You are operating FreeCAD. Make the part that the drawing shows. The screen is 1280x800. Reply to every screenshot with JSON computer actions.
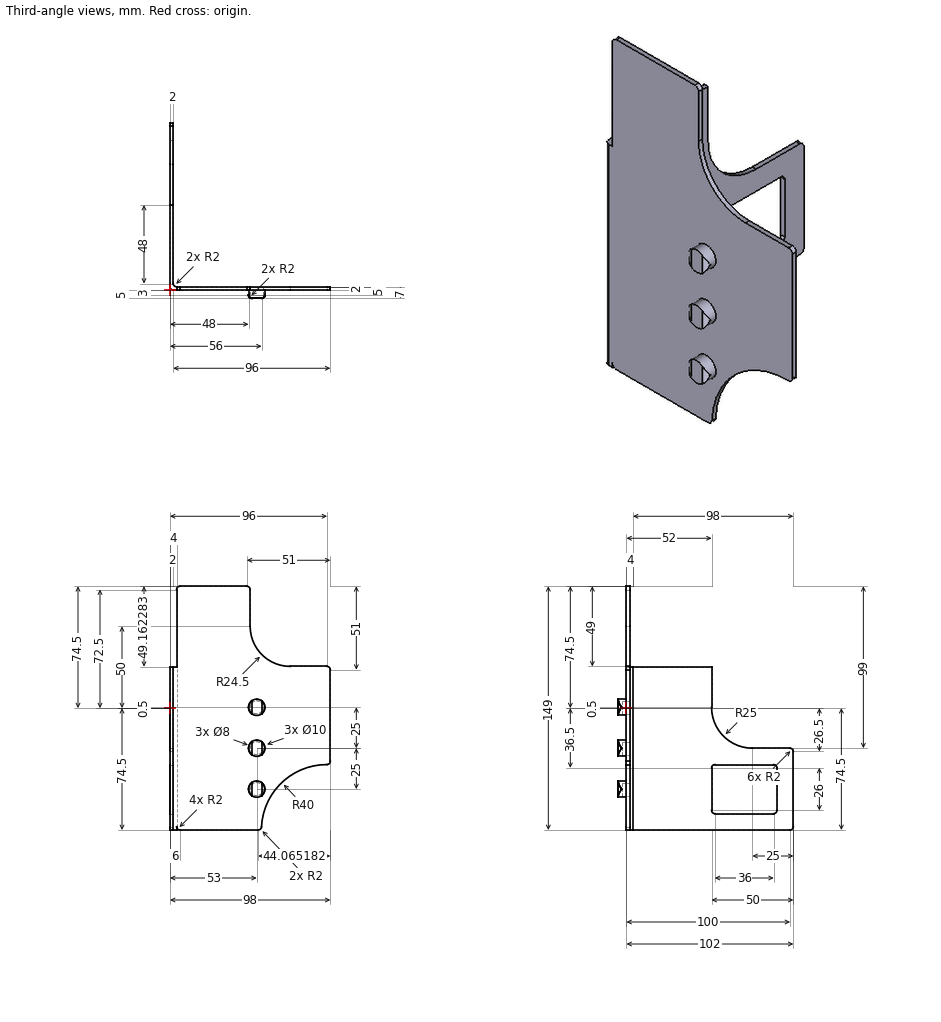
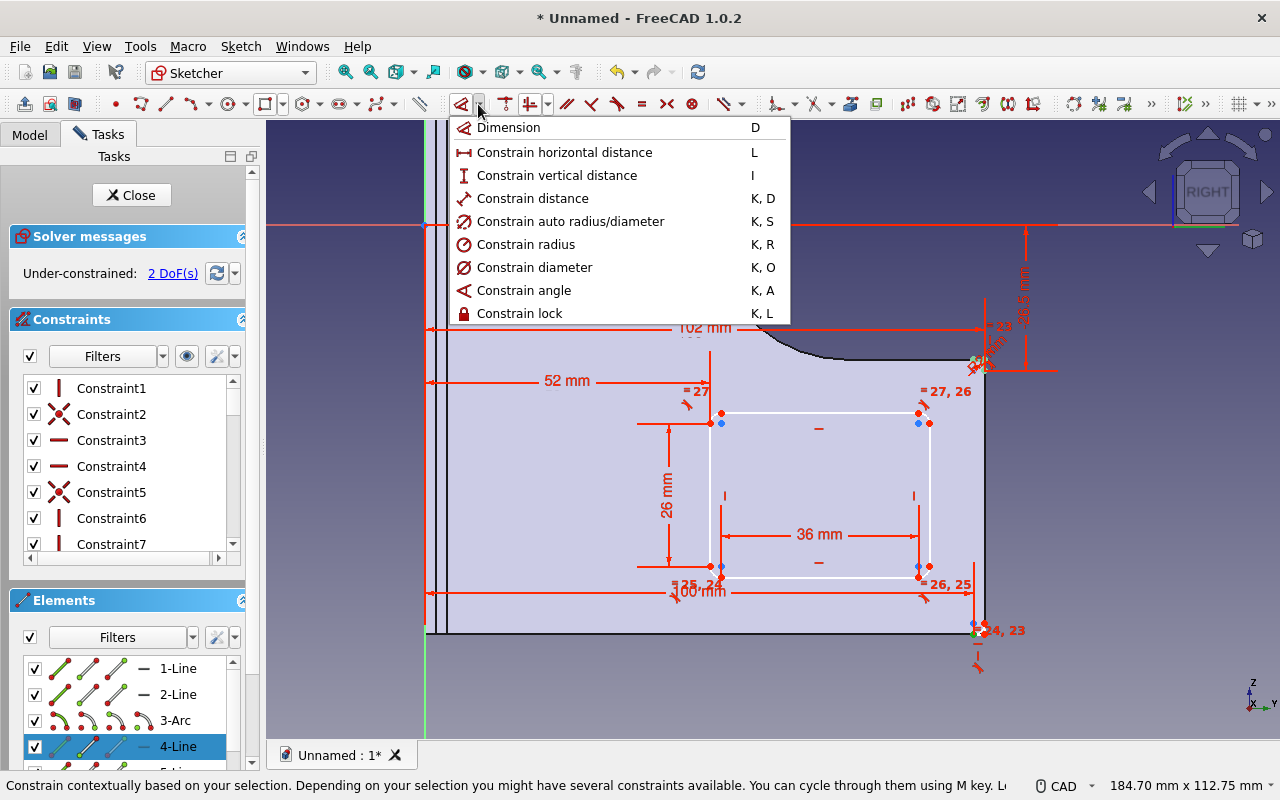
{"action": "left_click", "coordinate": [620, 176]}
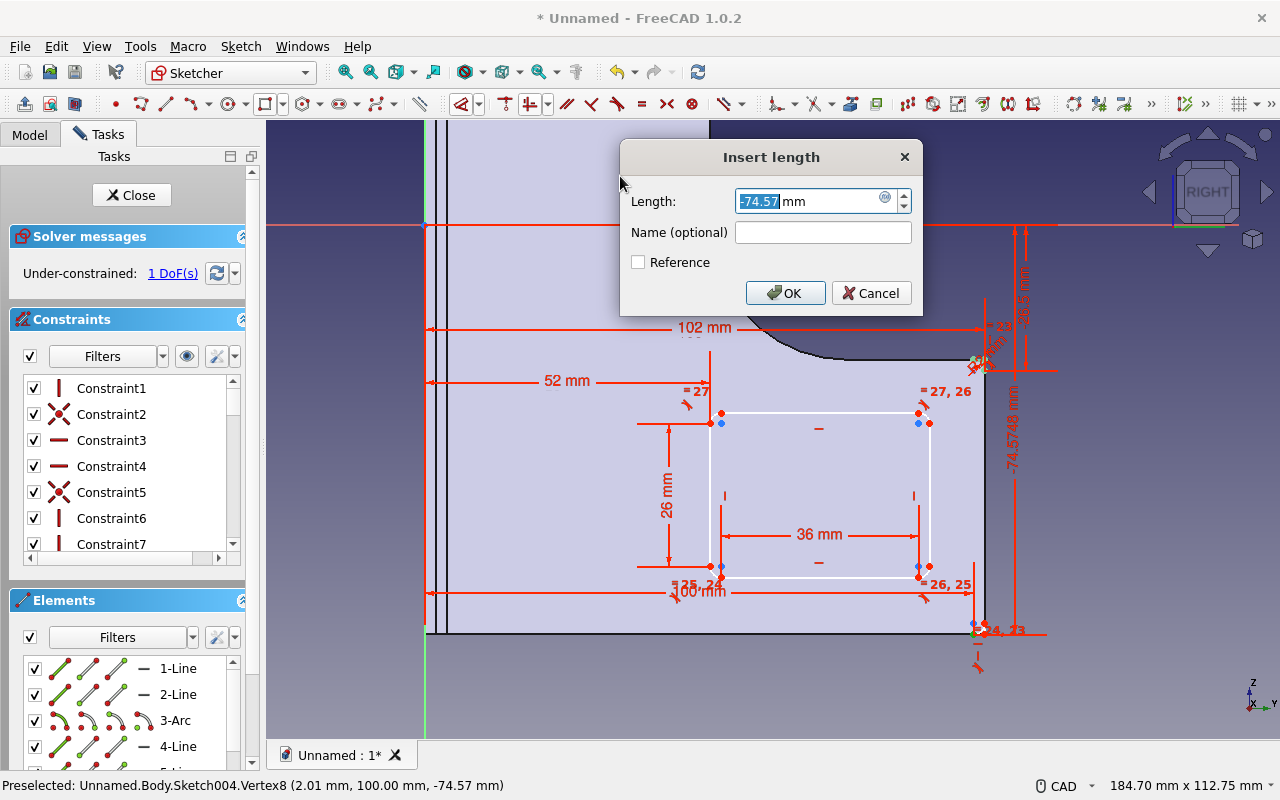
{"action": "type", "text": "-74.5"}
{"action": "key", "text": "Return"}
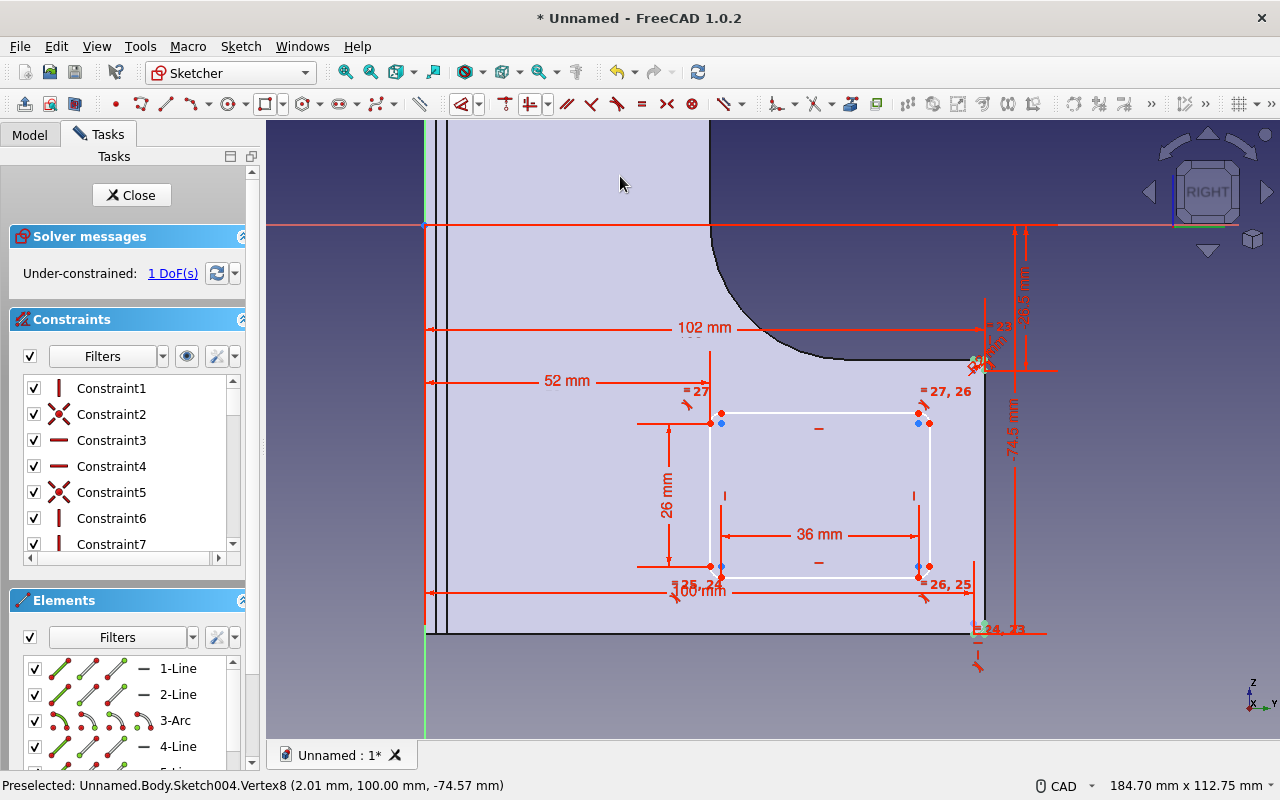
{"action": "left_click", "coordinate": [710, 424]}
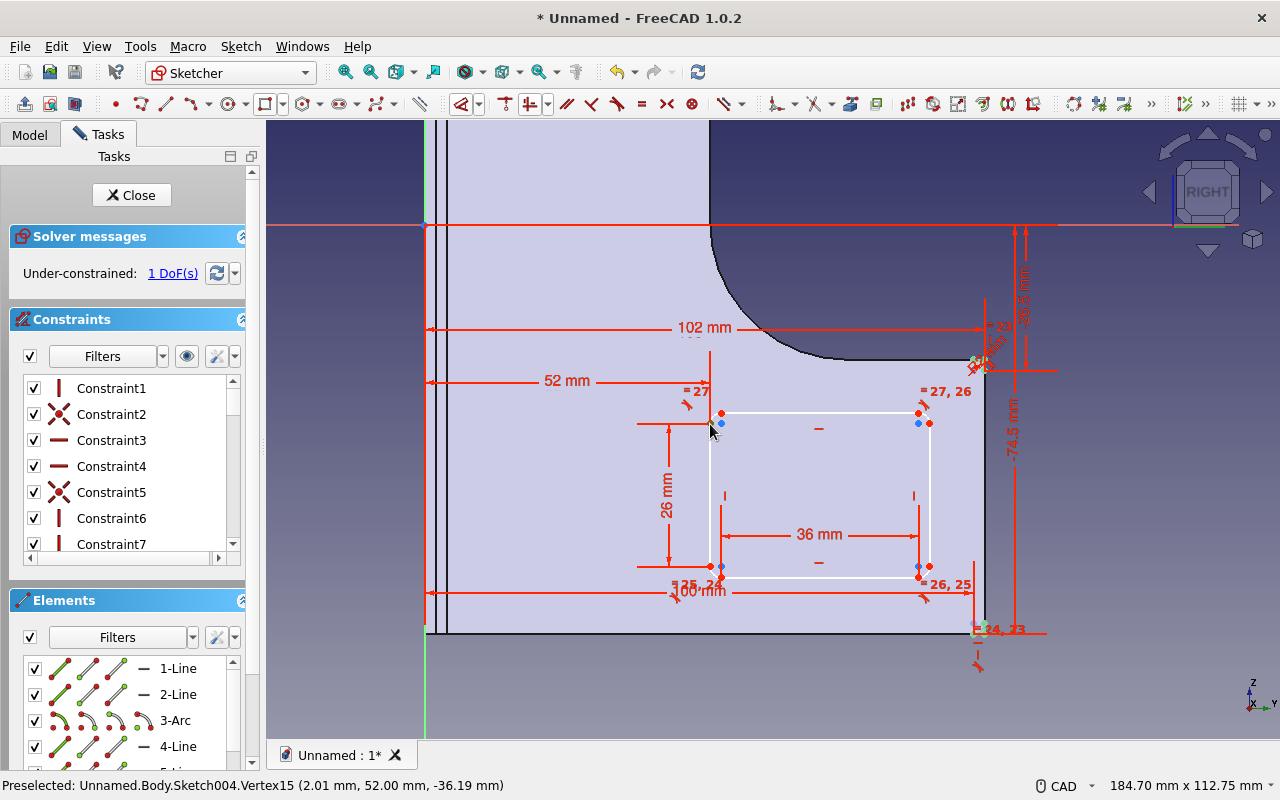
{"action": "left_click", "coordinate": [478, 104]}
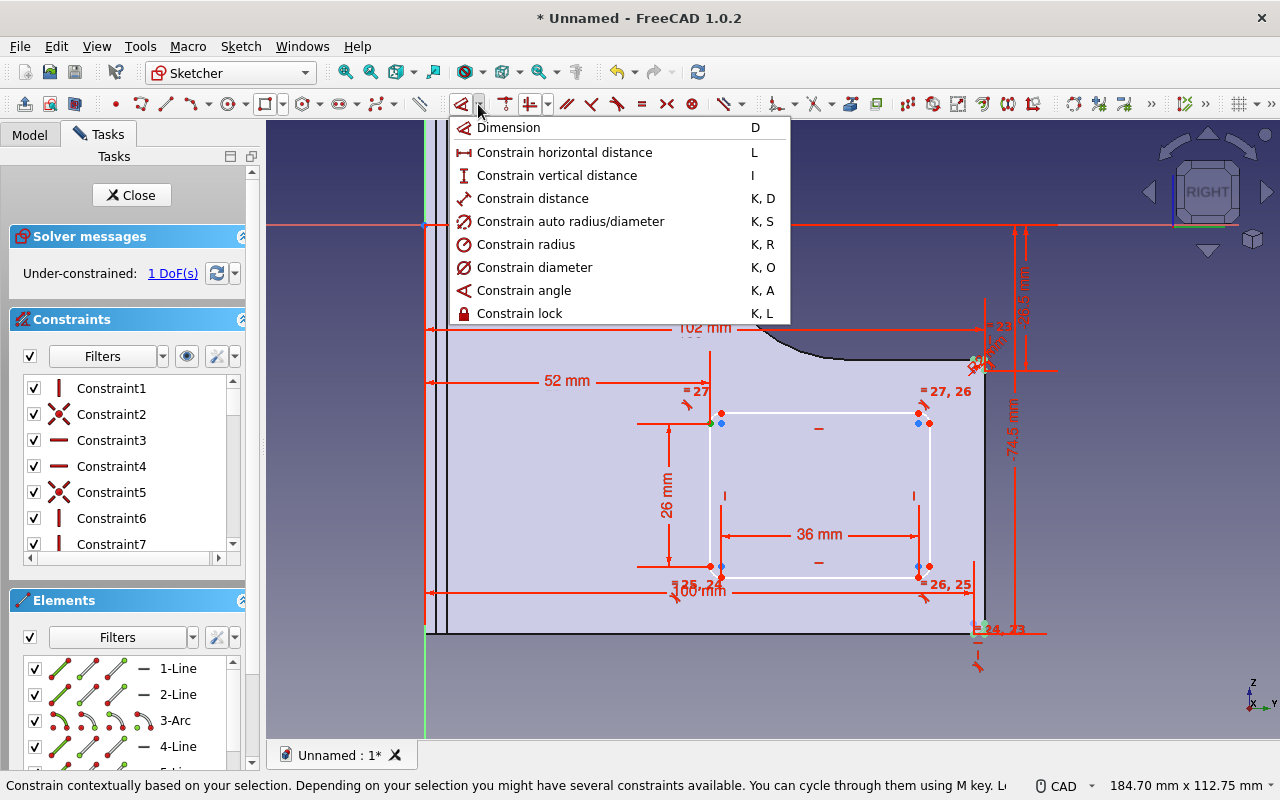
{"action": "left_click", "coordinate": [620, 176]}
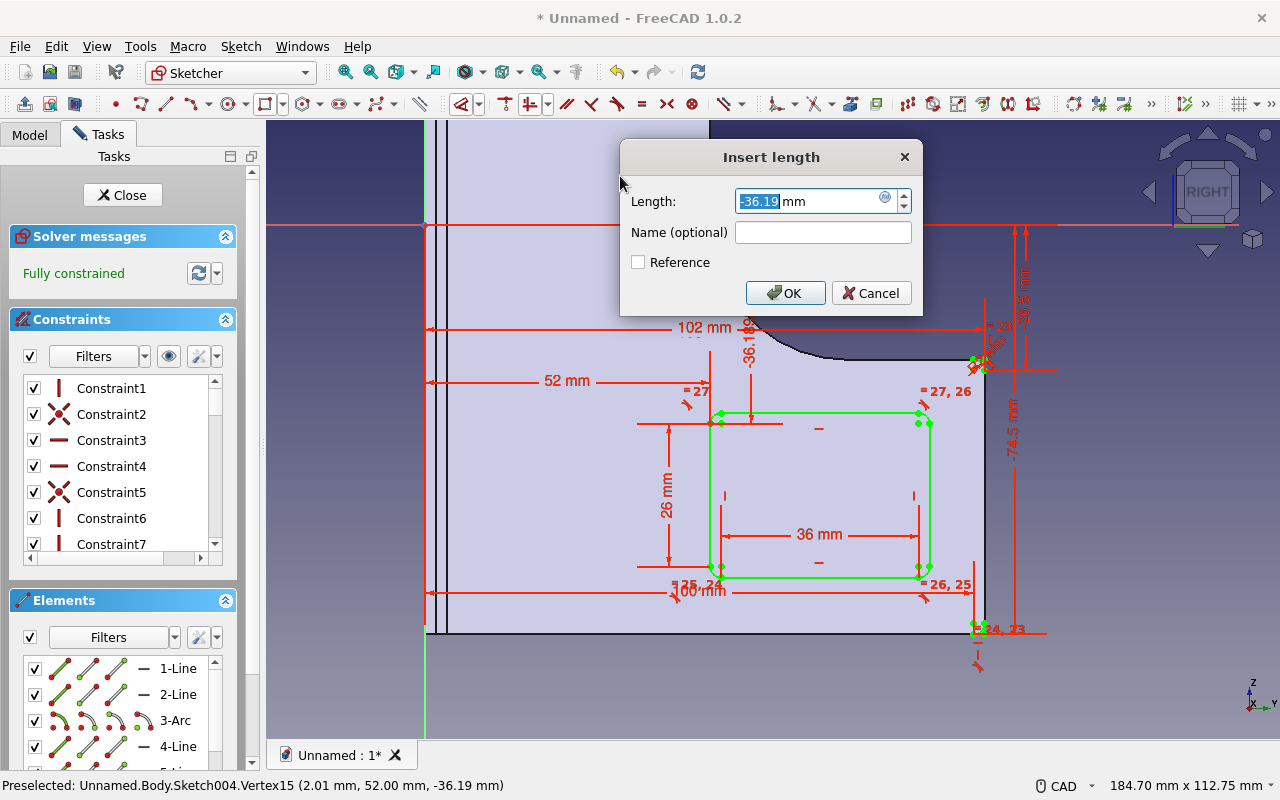
{"action": "type", "text": "-36.5"}
{"action": "key", "text": "Return"}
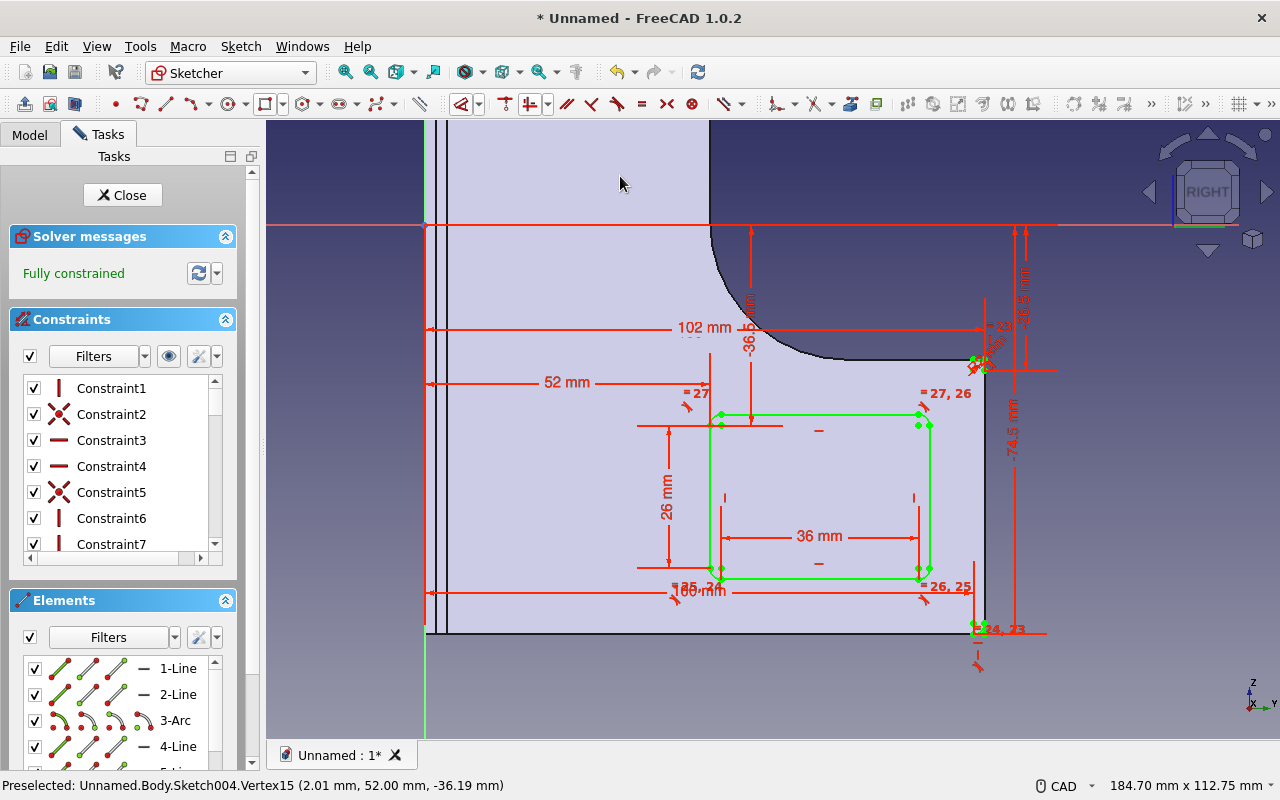
{"action": "left_click", "coordinate": [123, 195]}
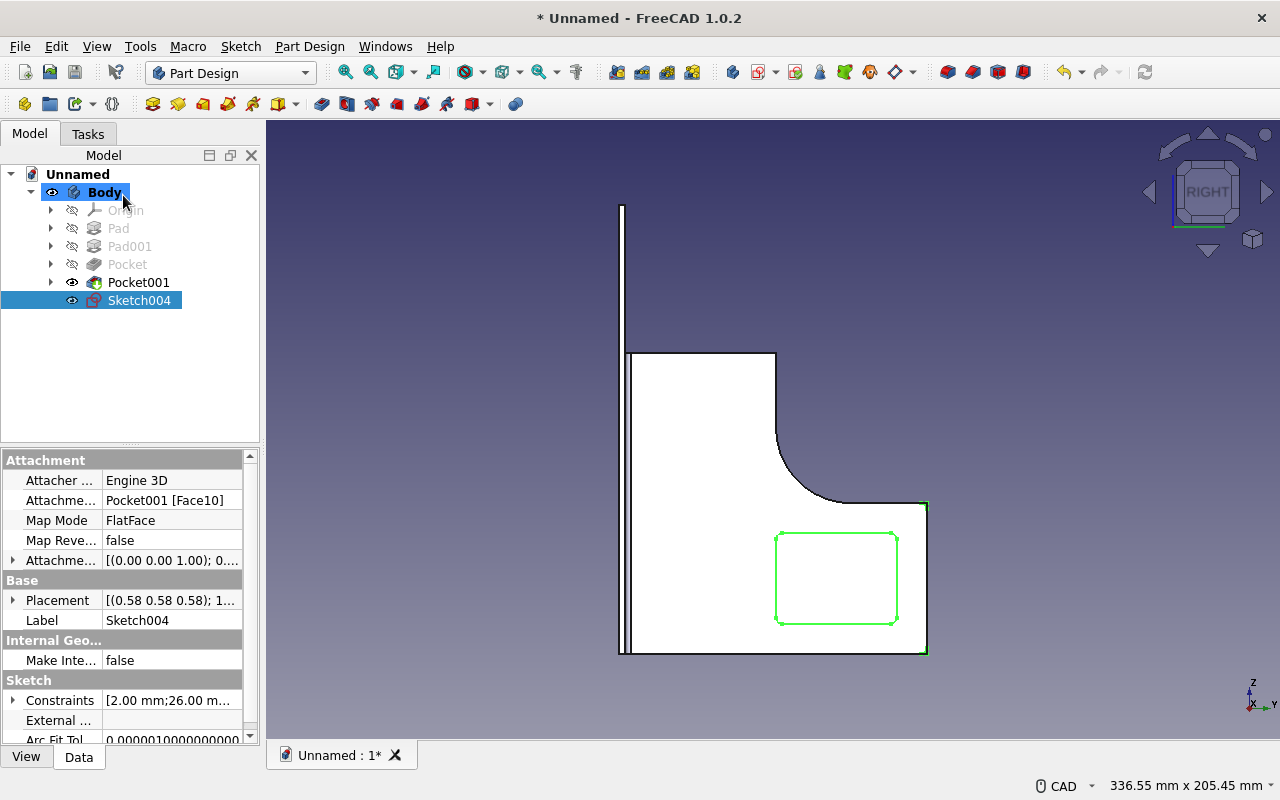
{"action": "left_click", "coordinate": [322, 104]}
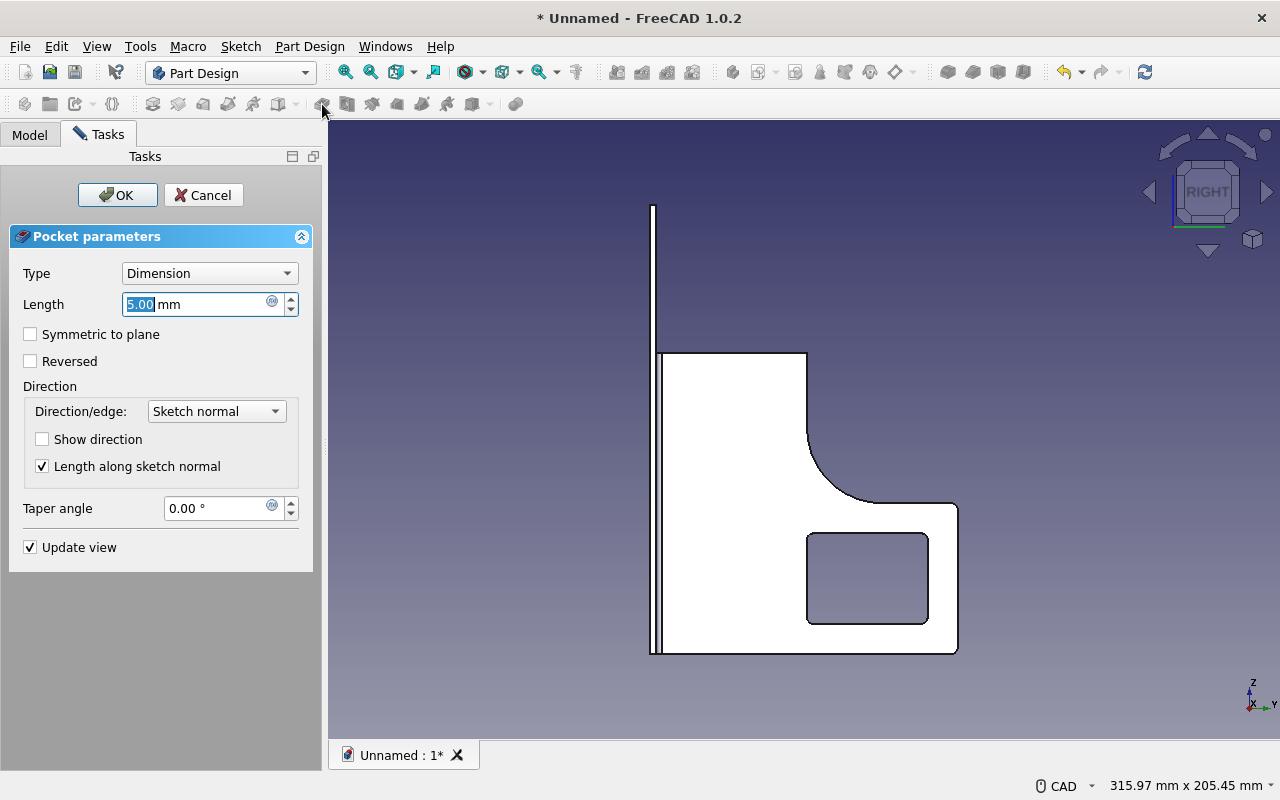
{"action": "type", "text": "2"}
{"action": "key", "text": "Tab"}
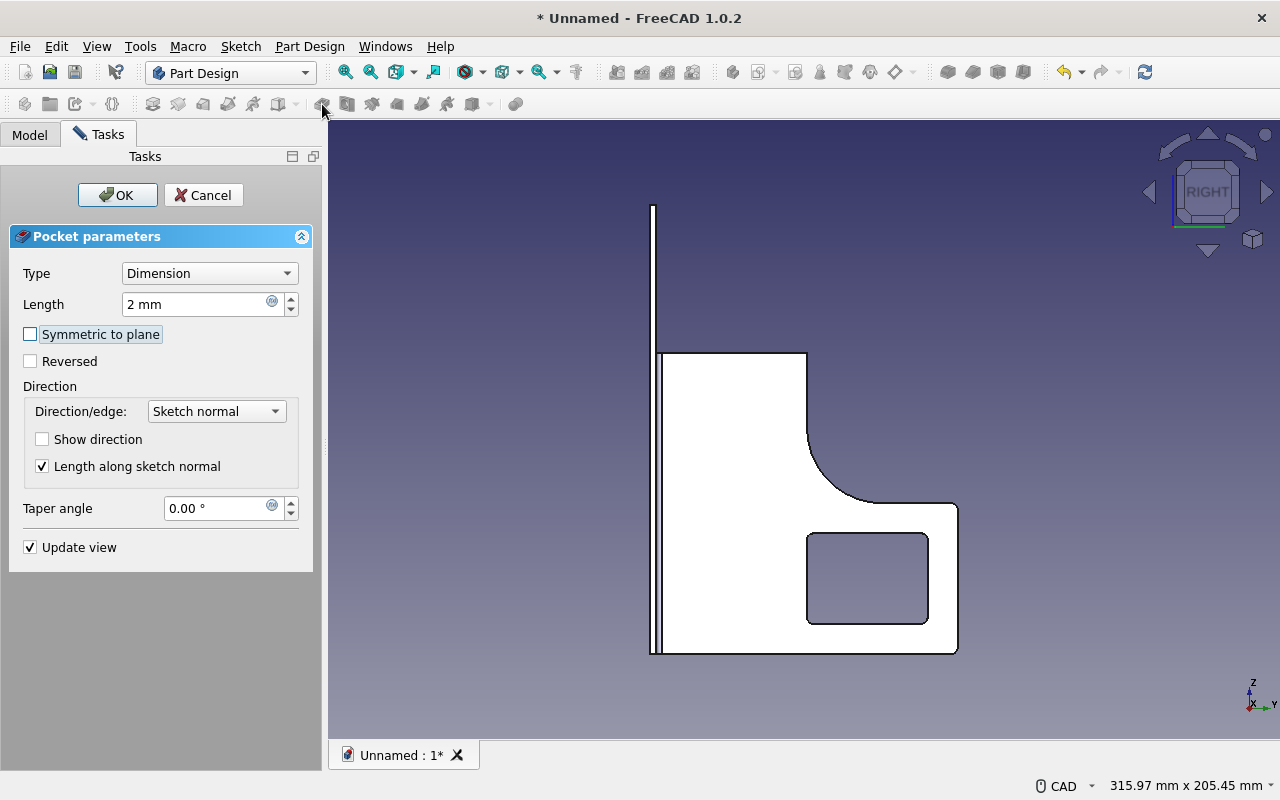
{"action": "left_click", "coordinate": [118, 195]}